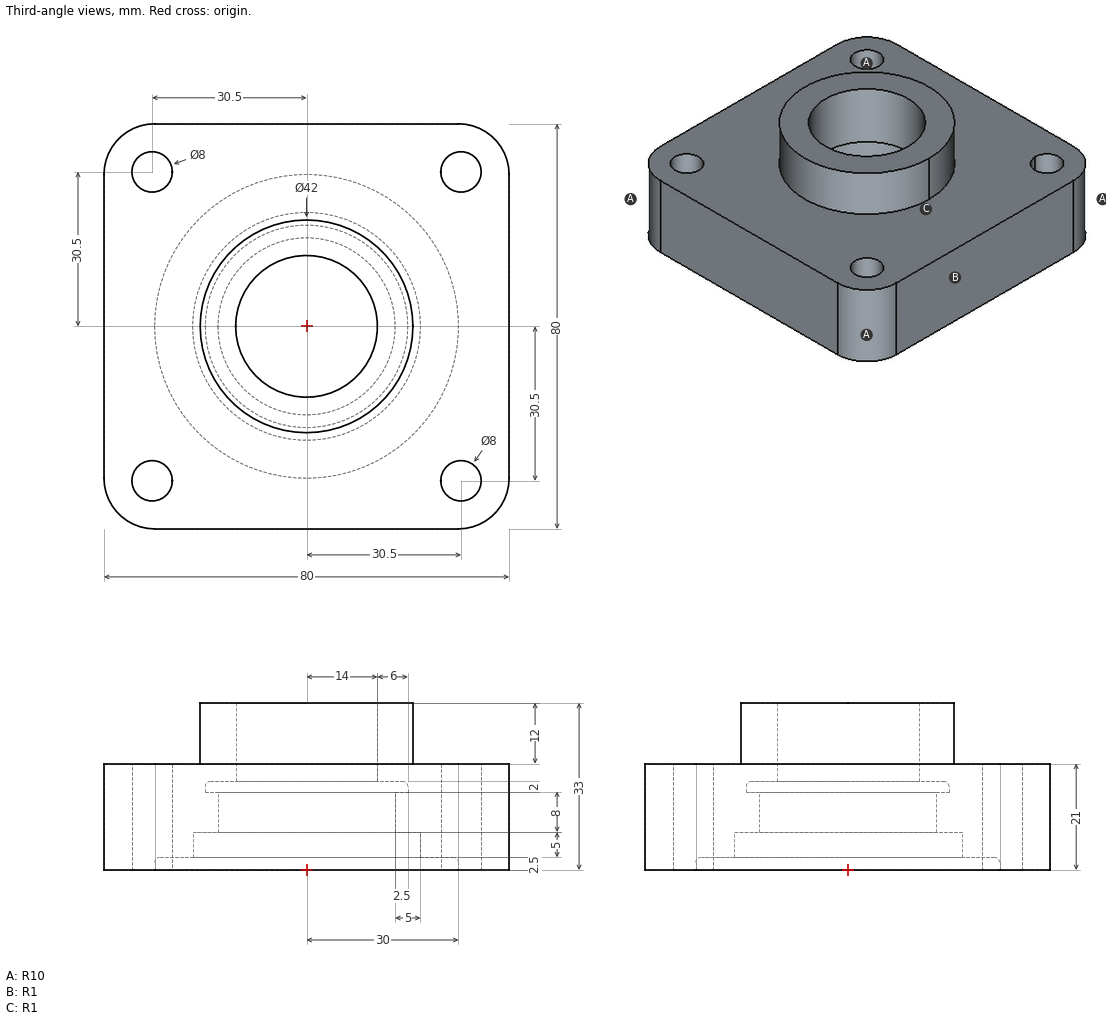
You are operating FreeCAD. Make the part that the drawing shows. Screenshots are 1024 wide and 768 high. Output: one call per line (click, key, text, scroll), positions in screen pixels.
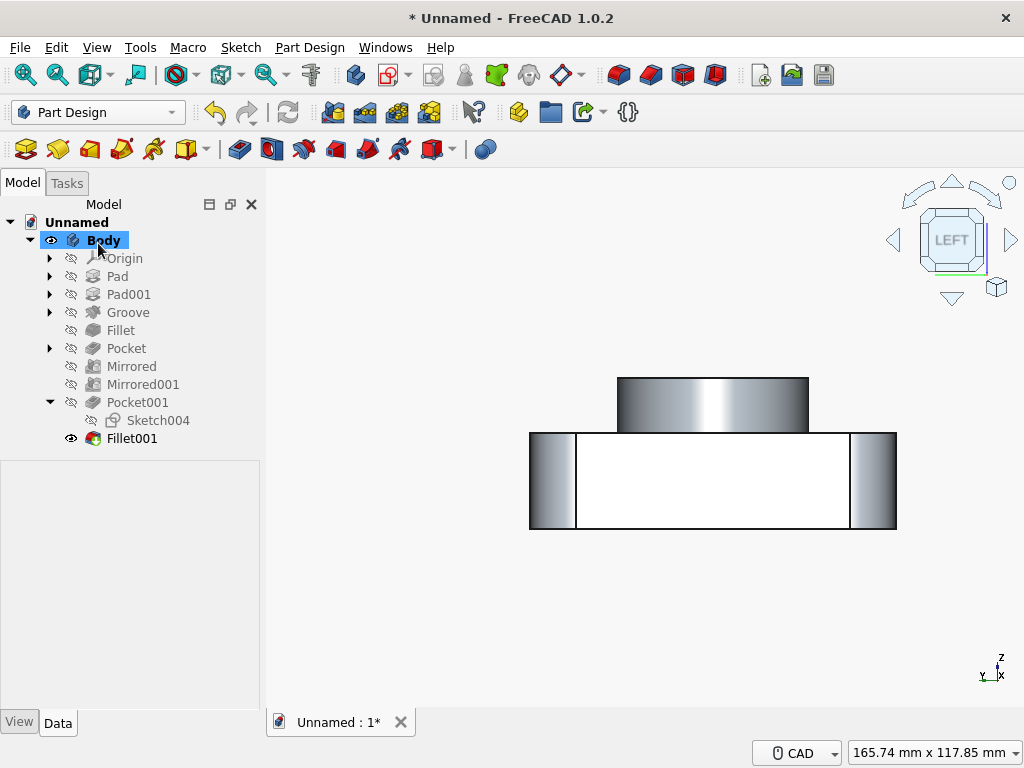
key(v)
key(3)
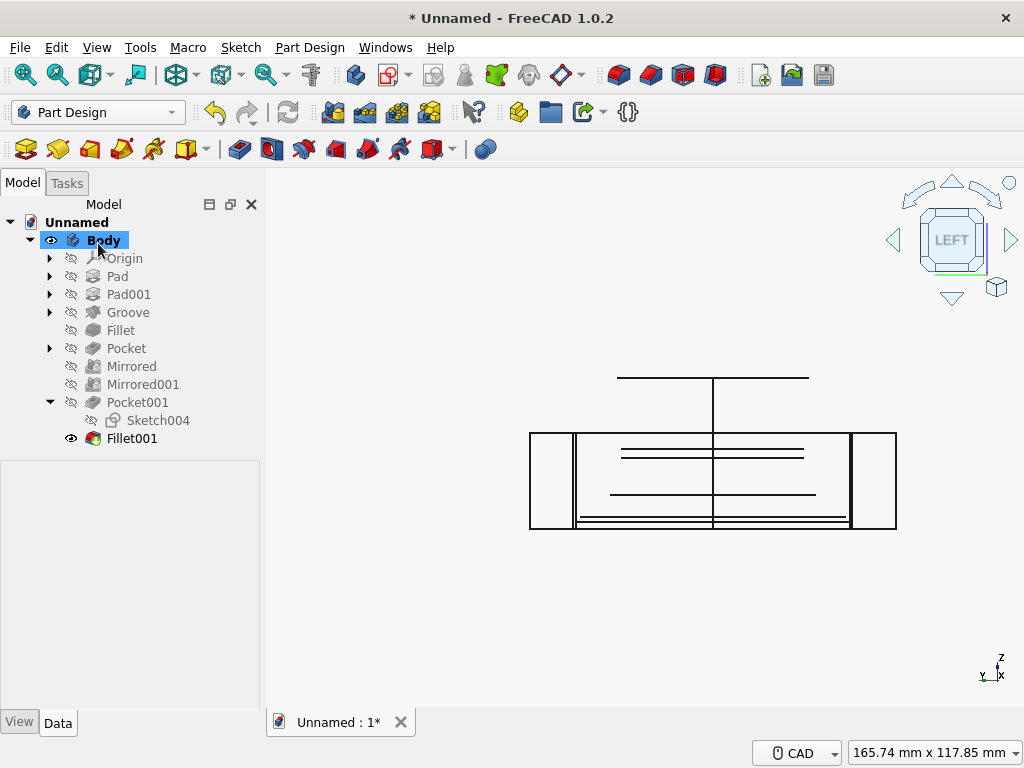
key(0)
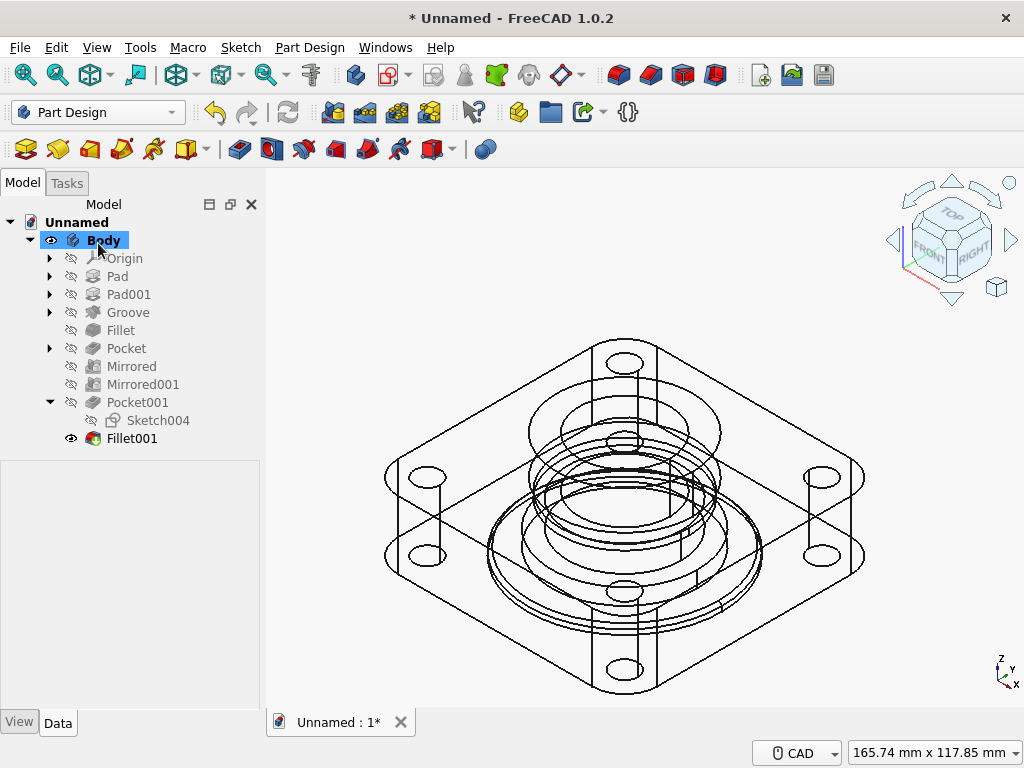
click(560, 452)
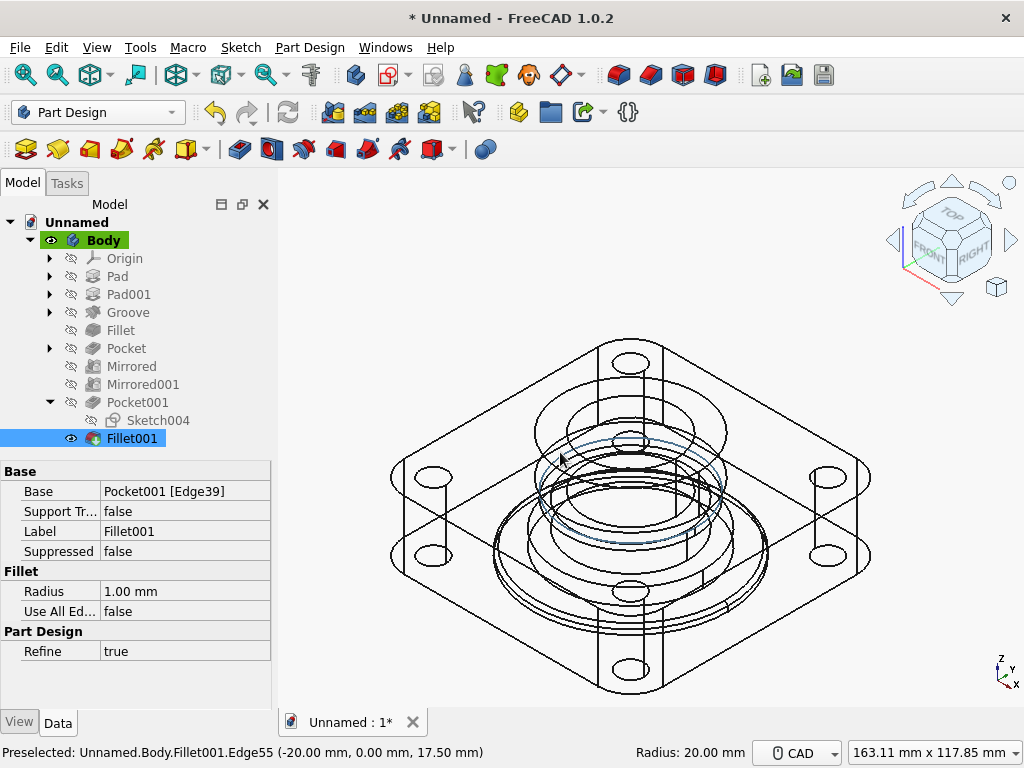
key(v)
key(1)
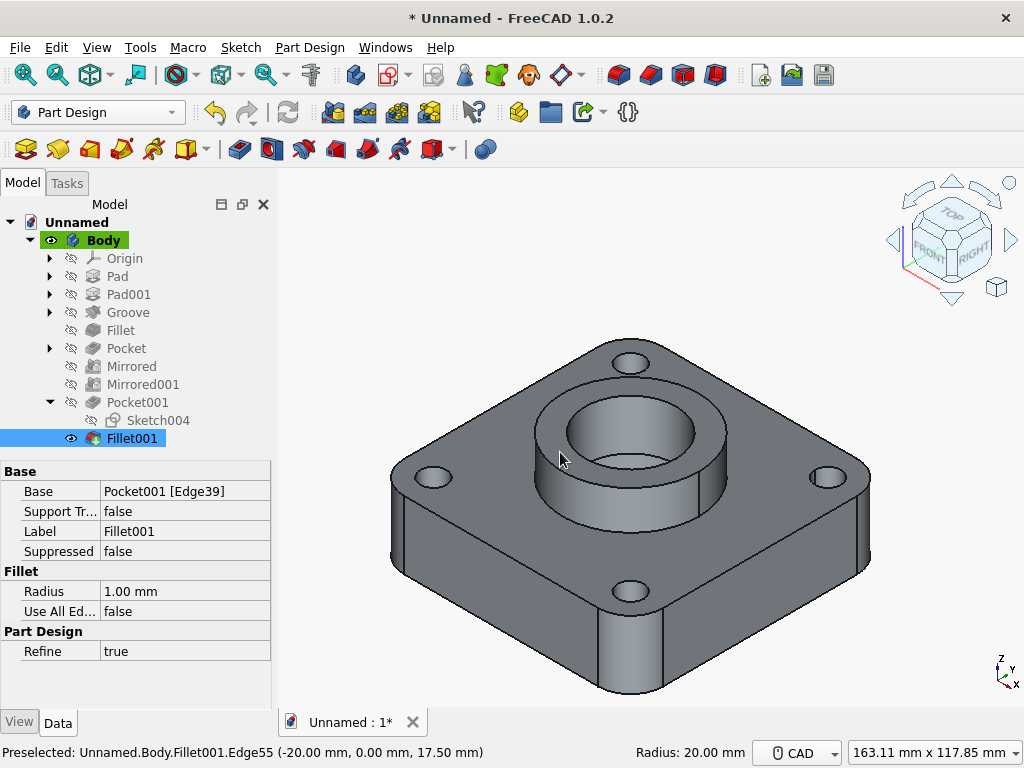
click(620, 76)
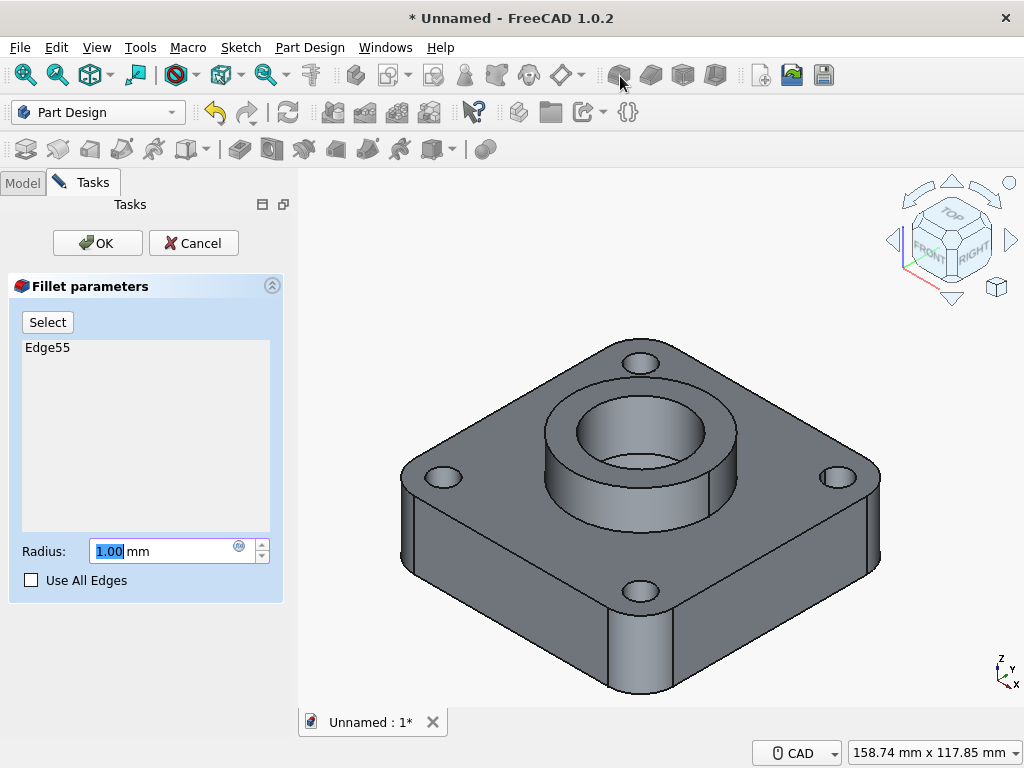
text(1)
key(Tab)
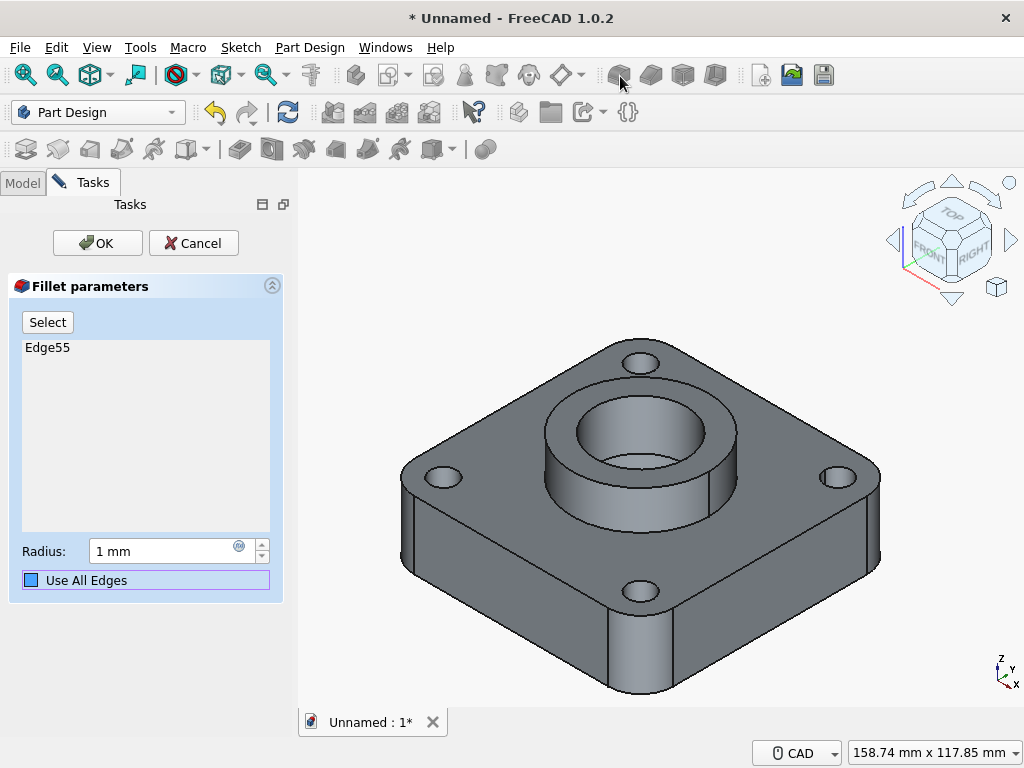
click(98, 243)